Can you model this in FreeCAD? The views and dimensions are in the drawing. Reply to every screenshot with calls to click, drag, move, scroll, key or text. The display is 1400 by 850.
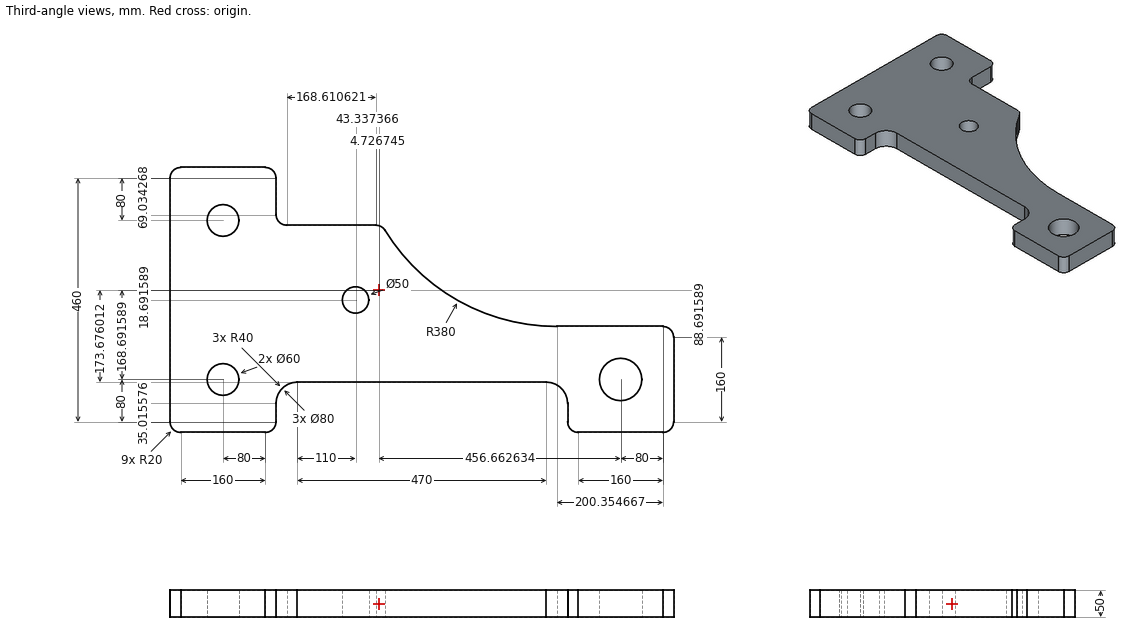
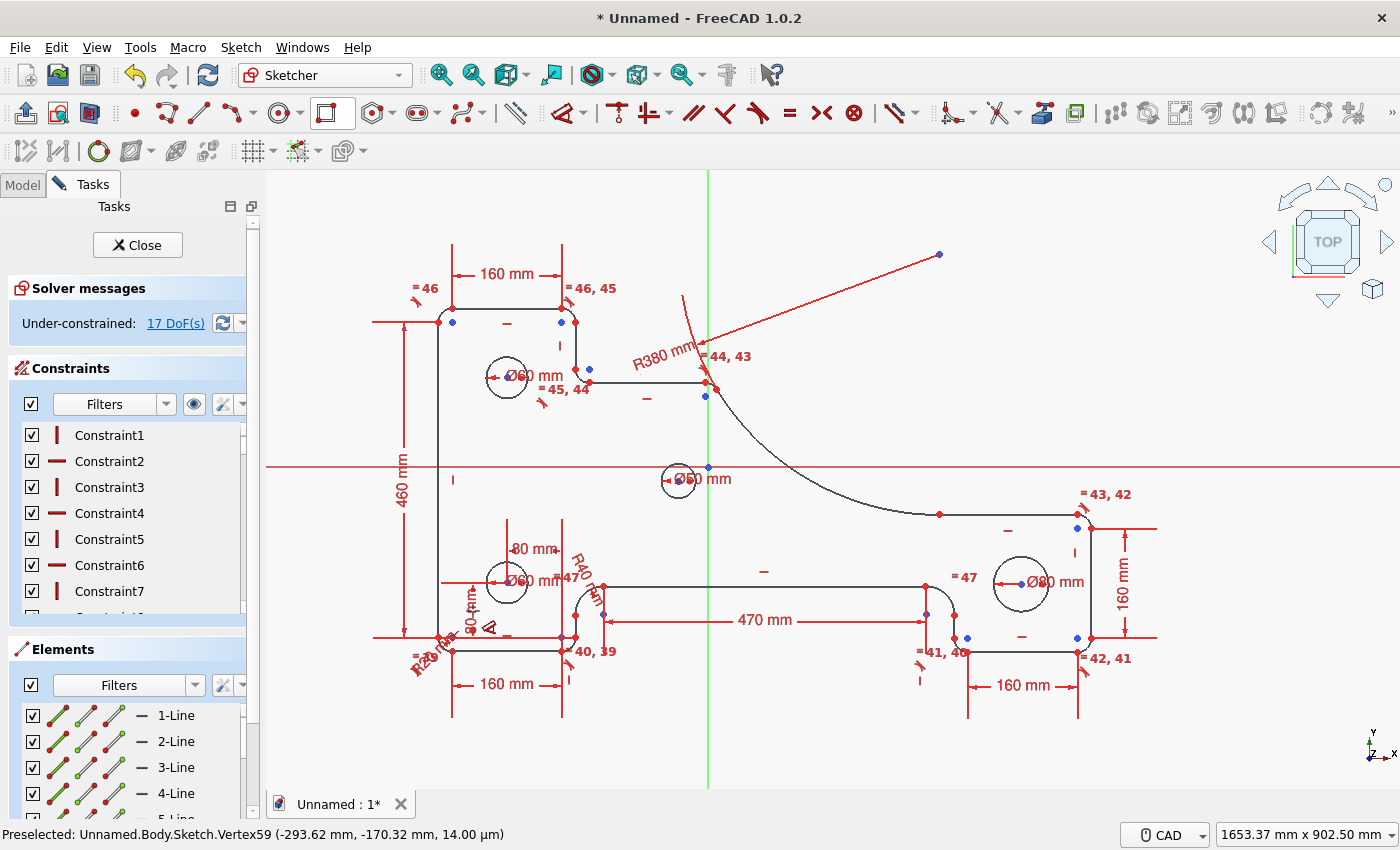
click(1078, 515)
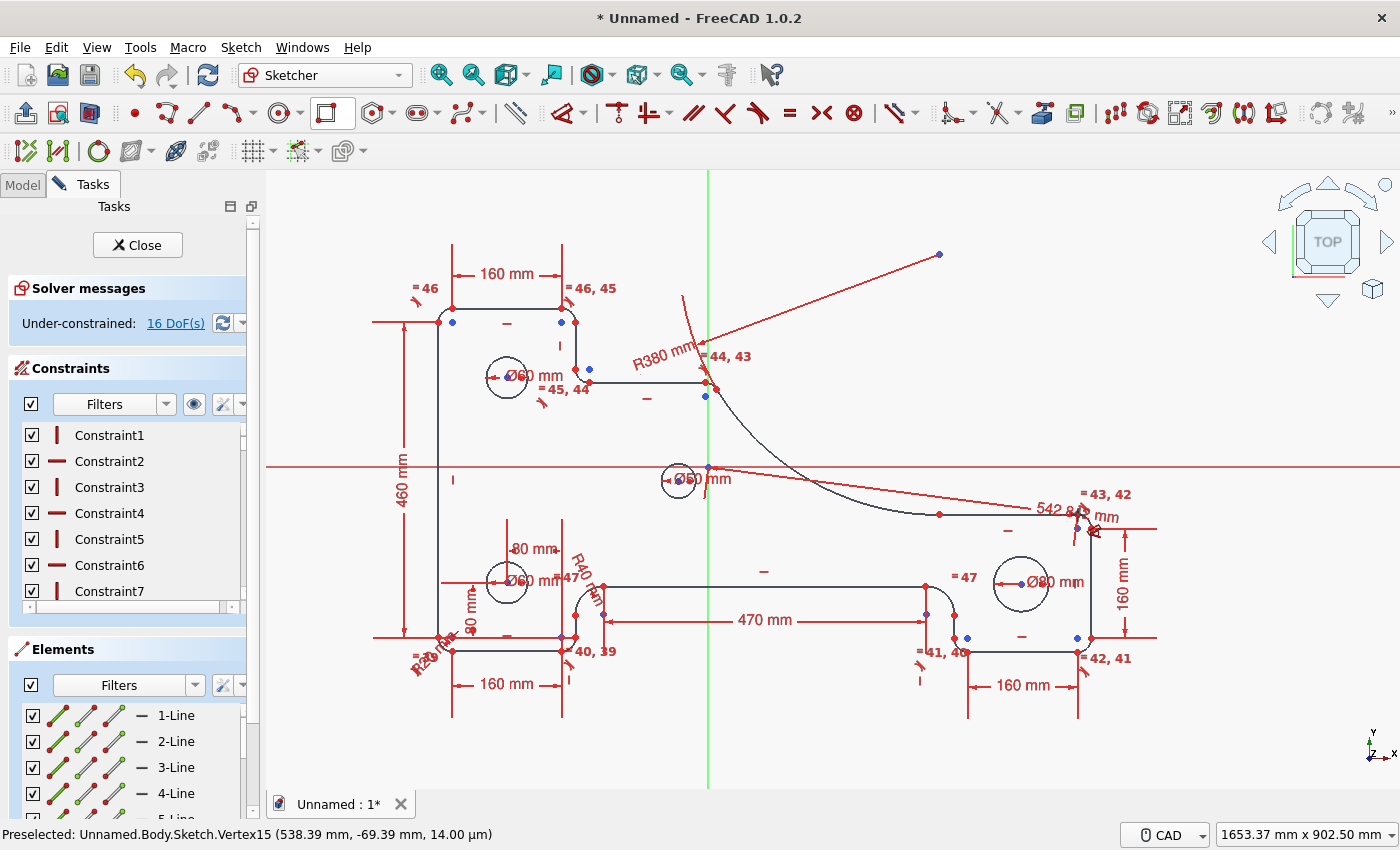
click(1021, 584)
click(1049, 618)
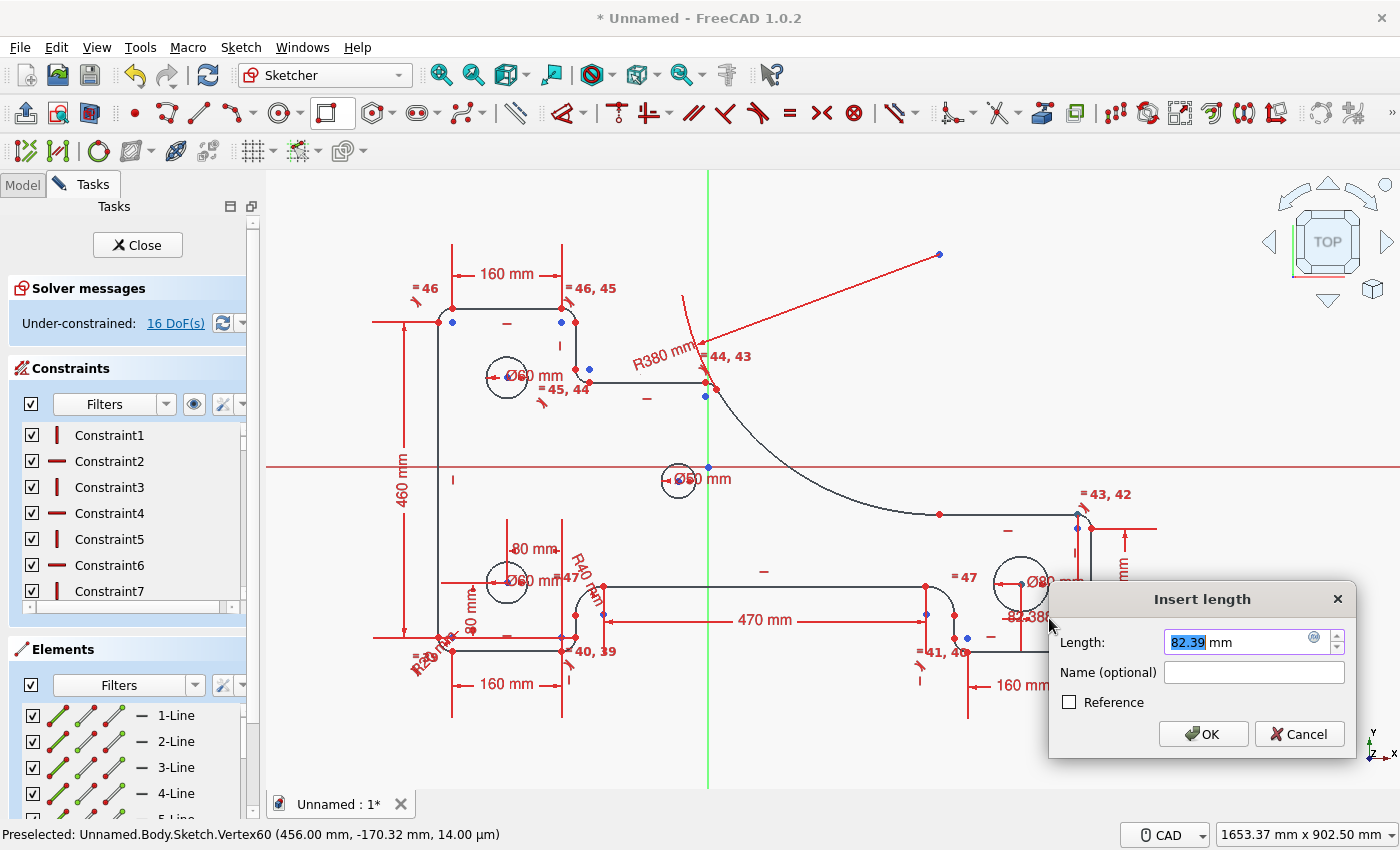
text(80)
key(Return)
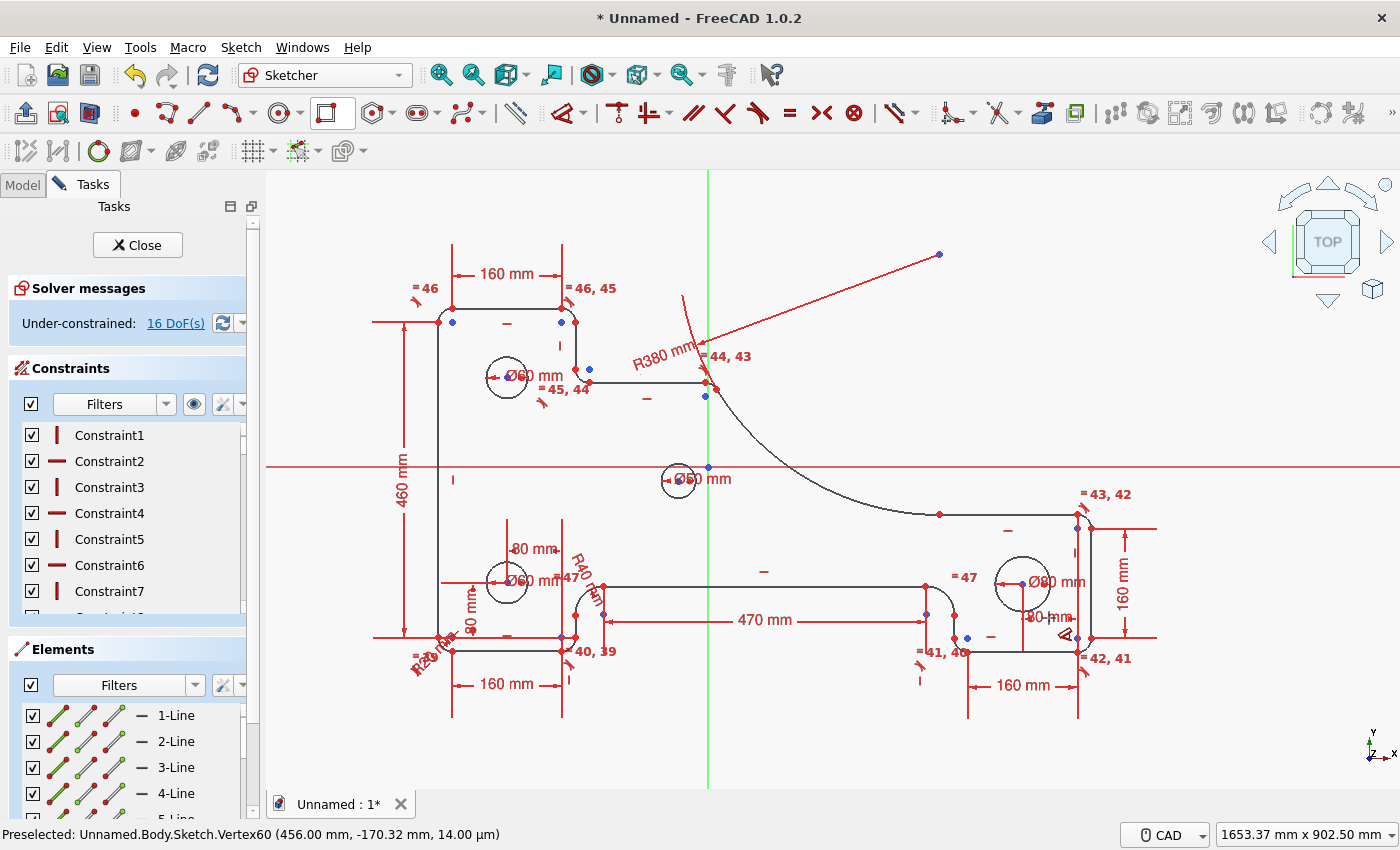
click(954, 638)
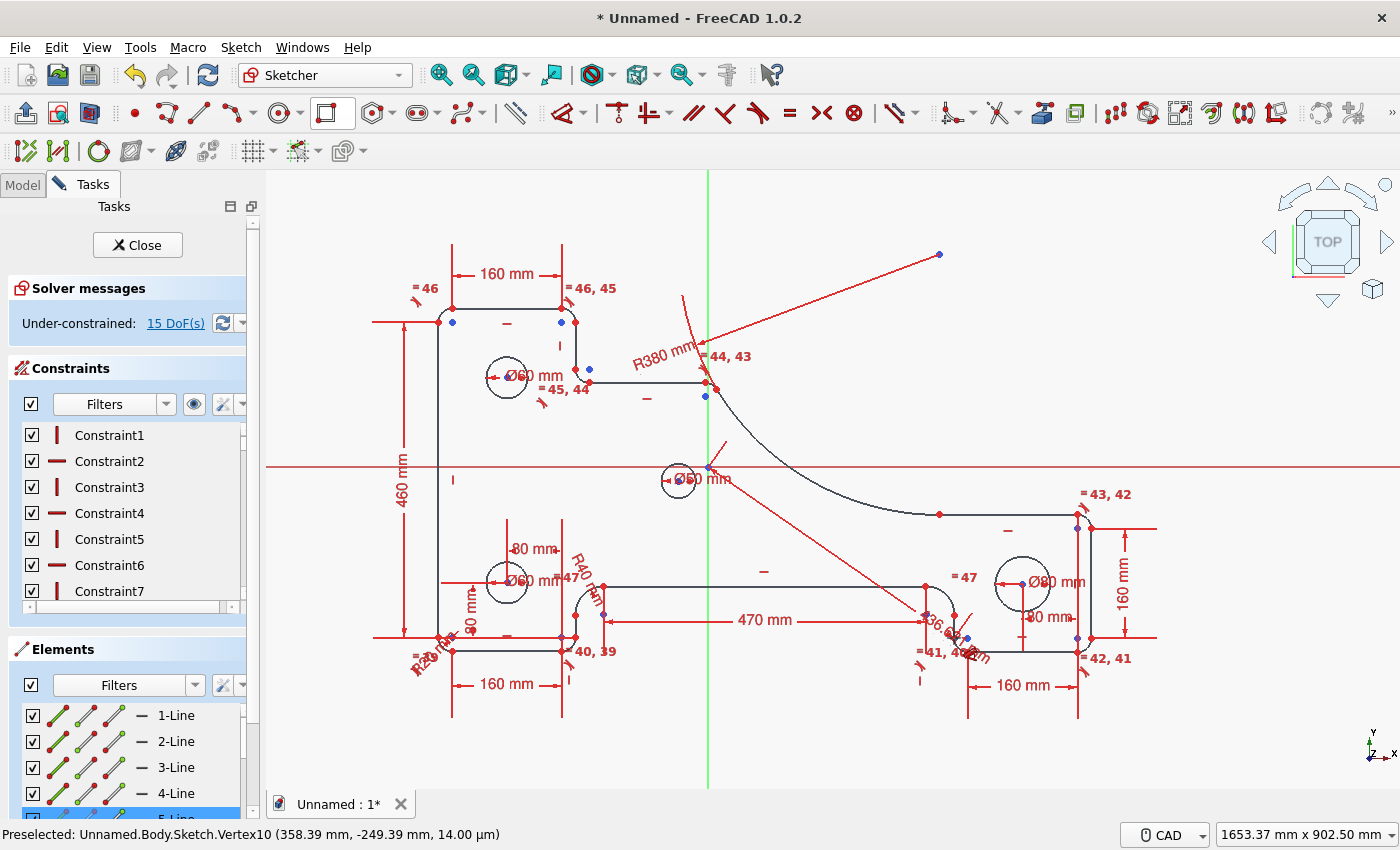
click(1023, 584)
click(920, 611)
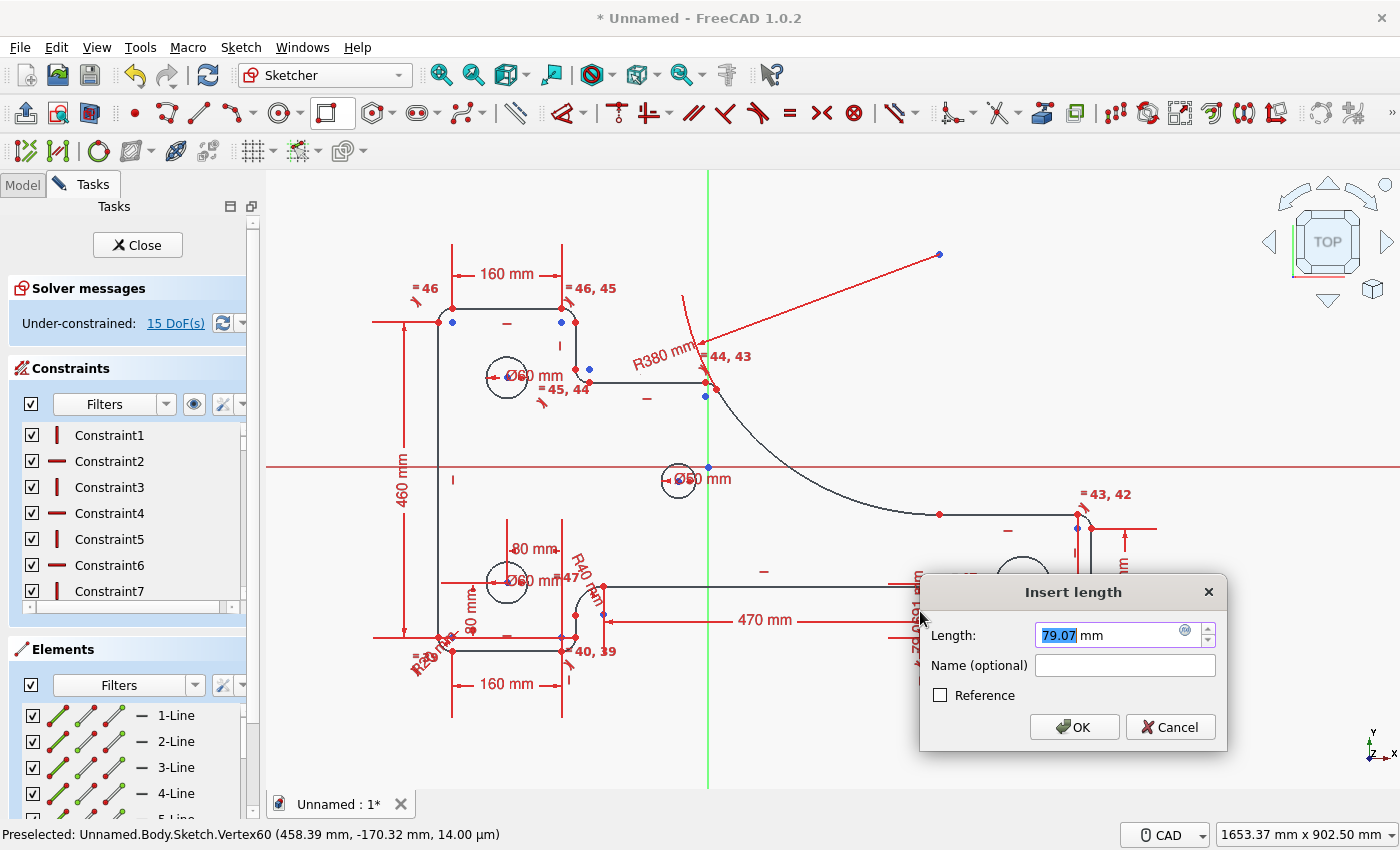
text(80)
key(Return)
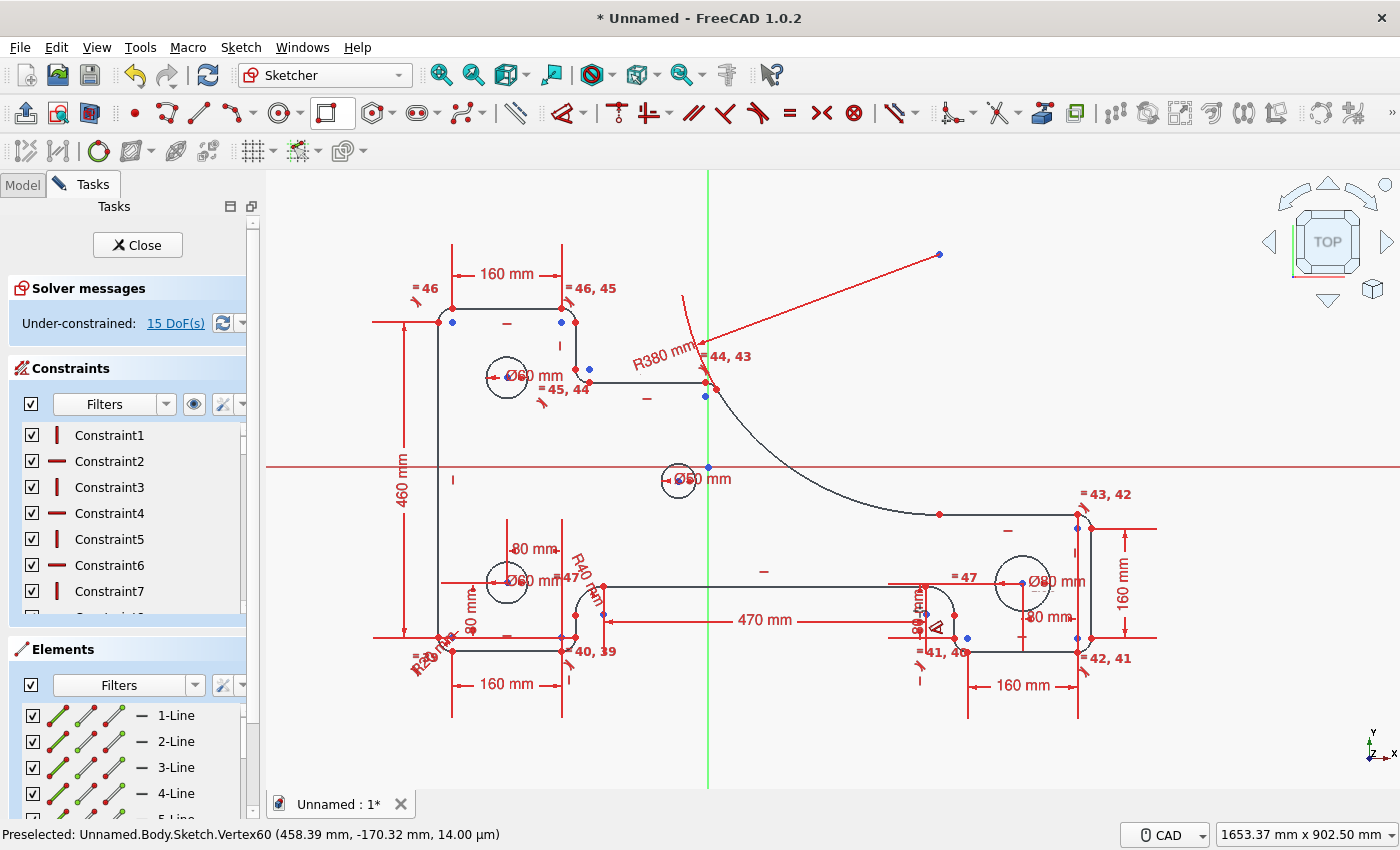
click(562, 309)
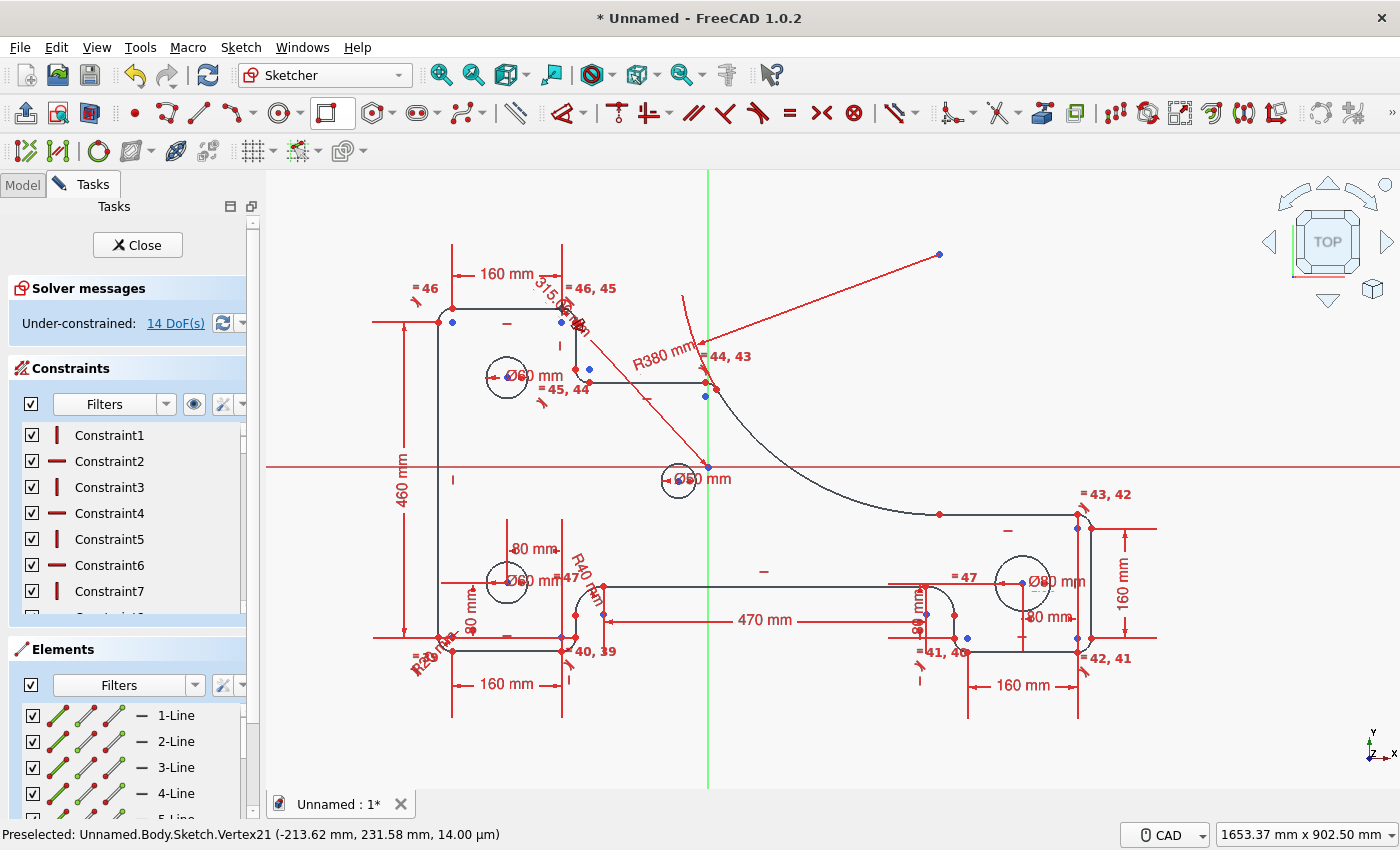
click(507, 378)
click(534, 412)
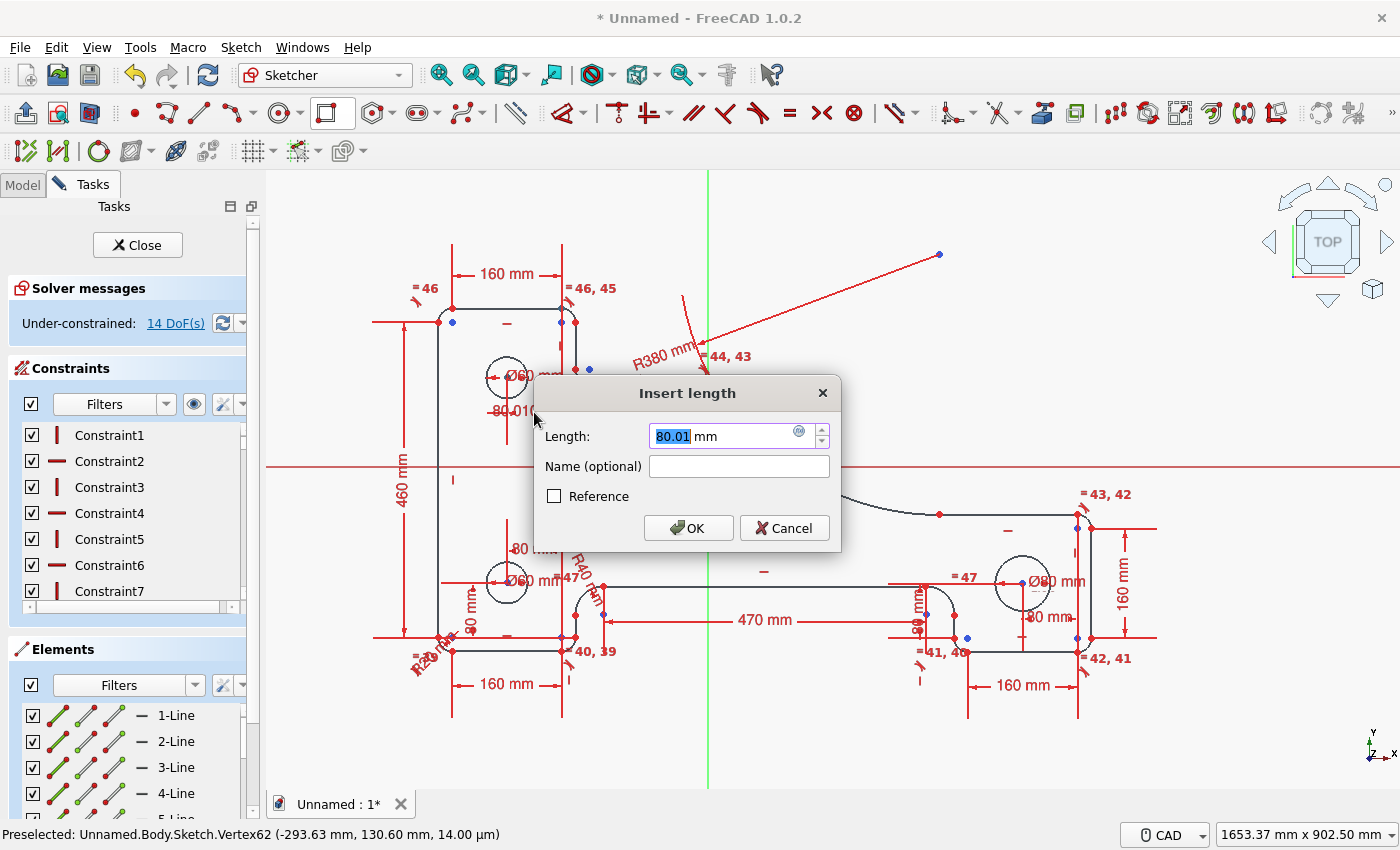
text(80)
key(Return)